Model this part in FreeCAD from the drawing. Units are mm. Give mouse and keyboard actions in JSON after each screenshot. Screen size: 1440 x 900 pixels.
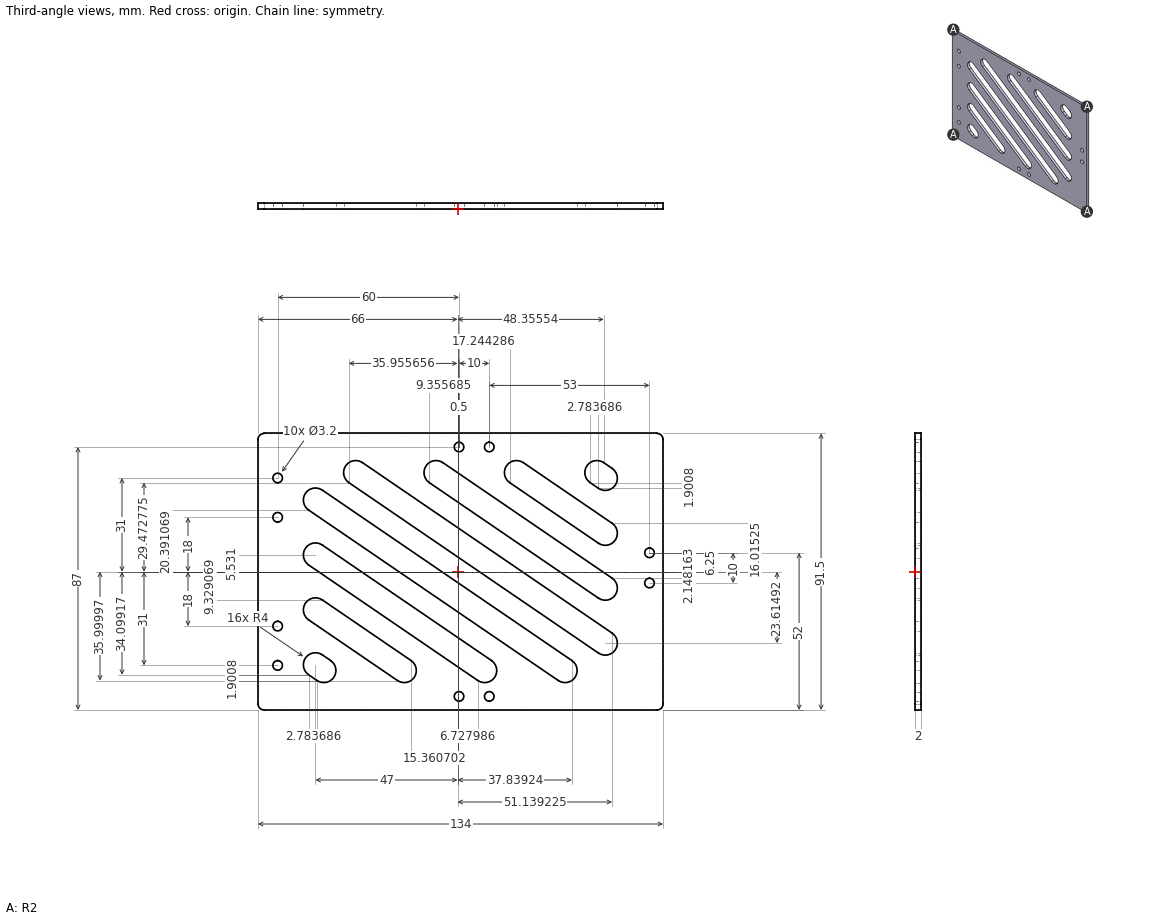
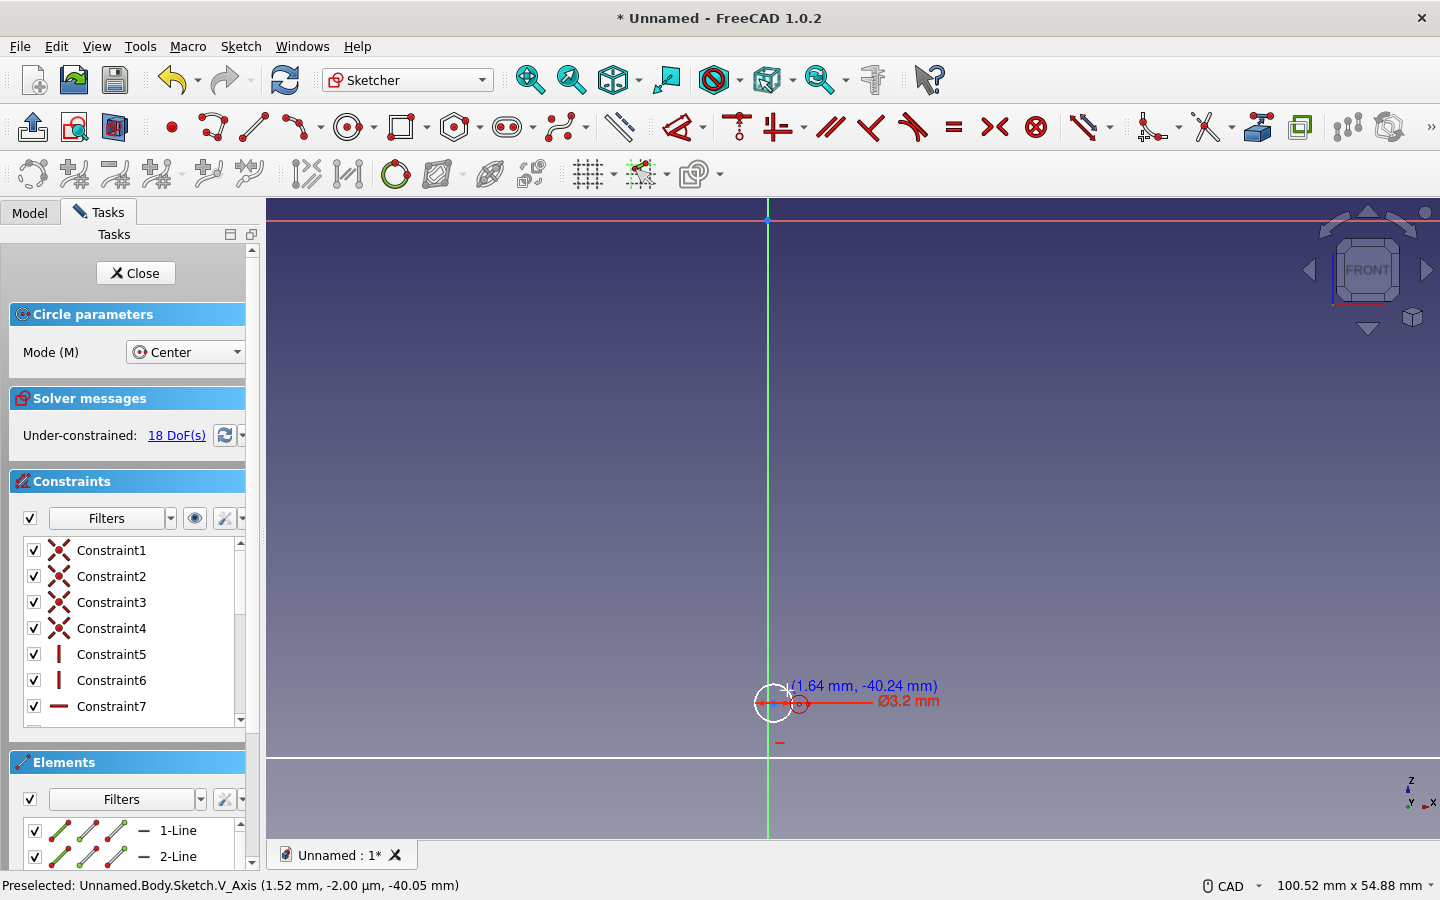
{"action": "scroll", "coordinate": [787, 692], "scroll_direction": "down", "scroll_amount": 5}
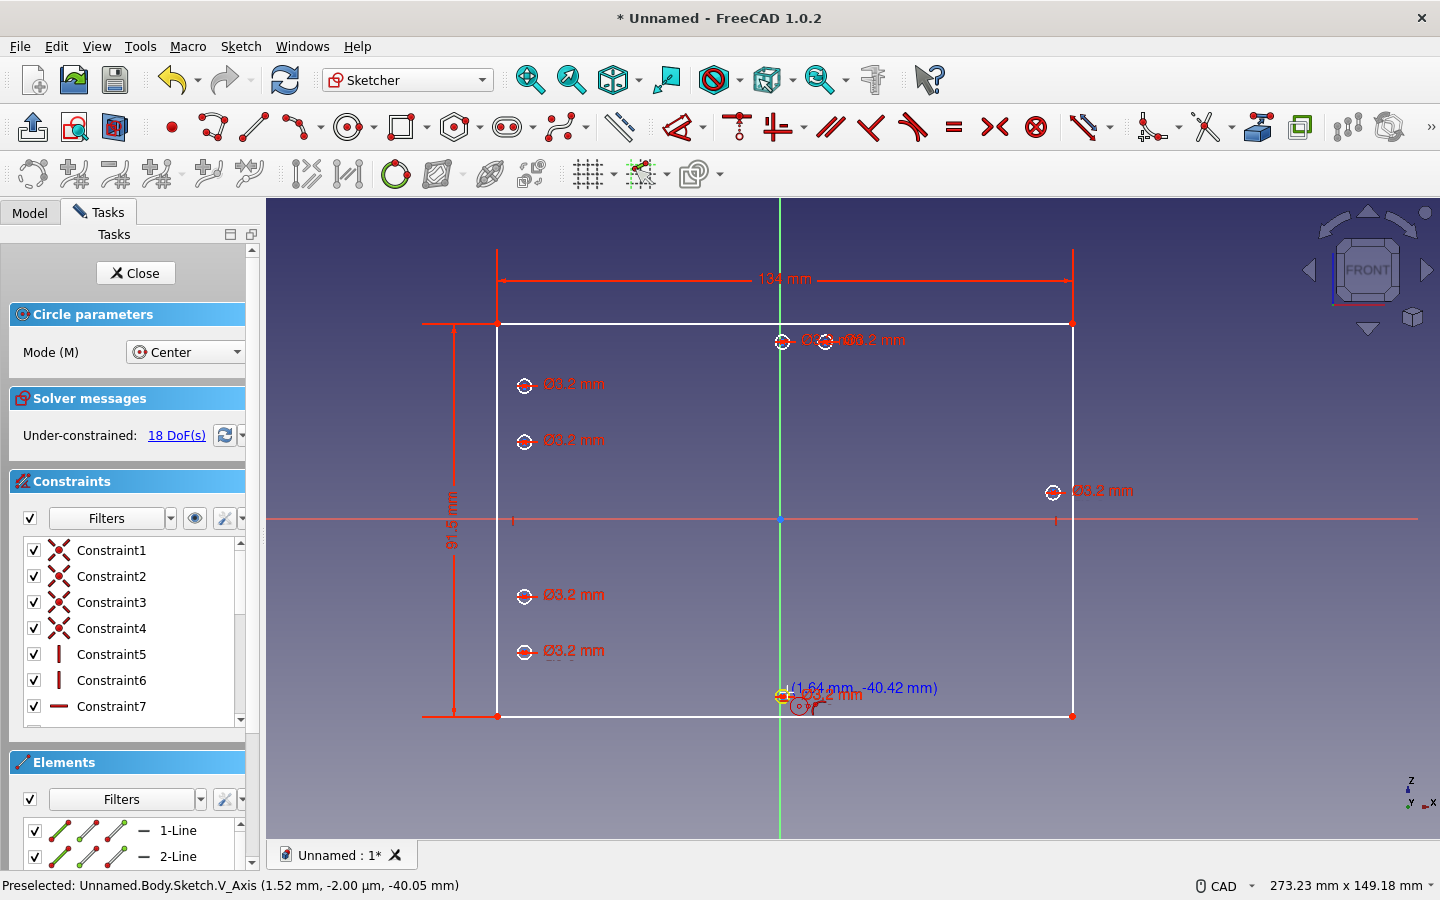
{"action": "scroll", "coordinate": [1053, 535], "scroll_direction": "up", "scroll_amount": 6}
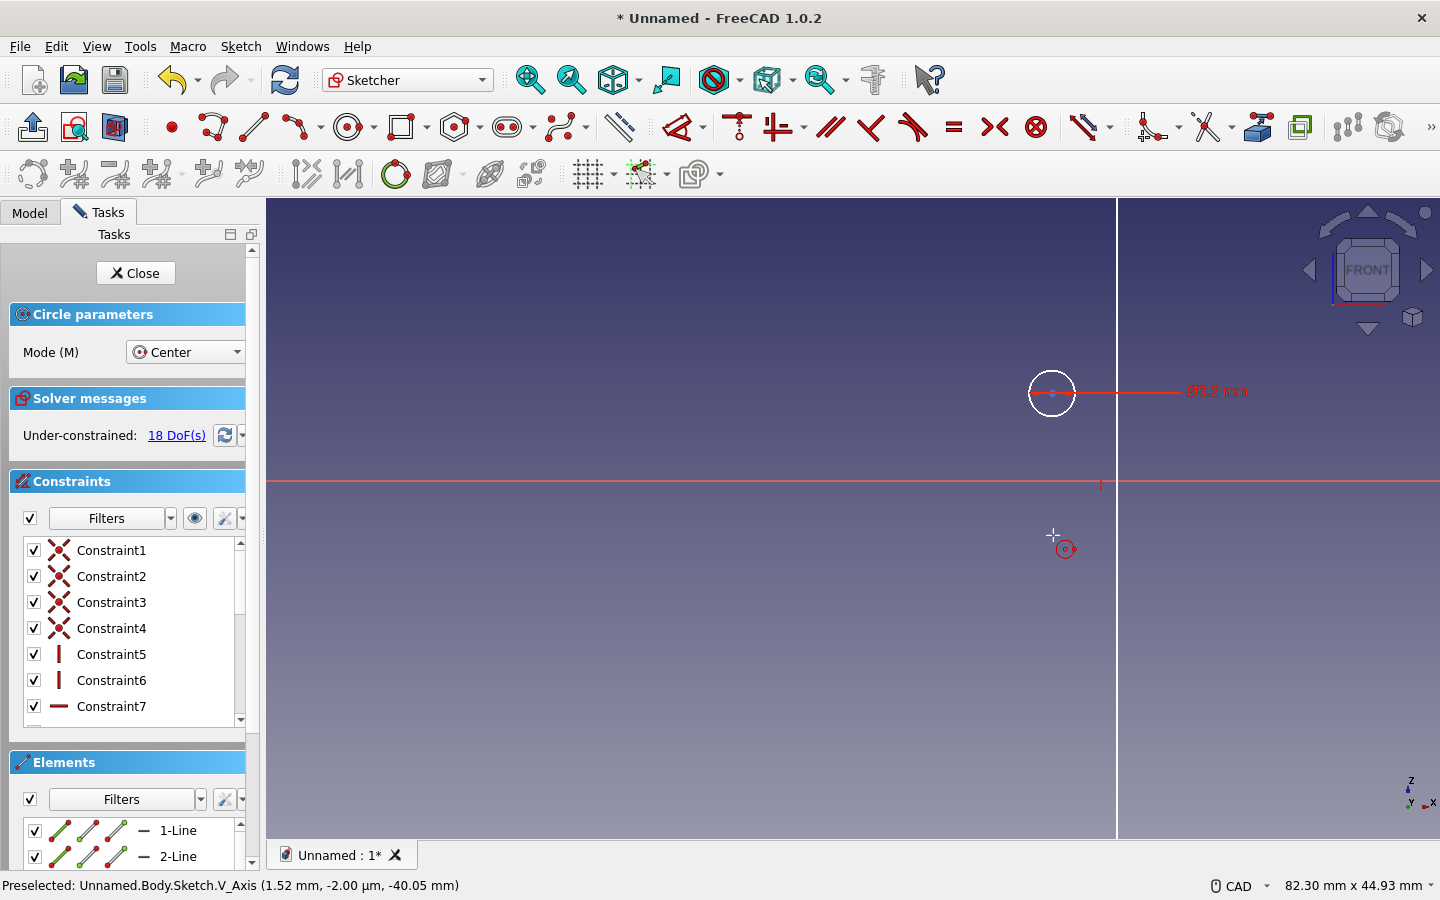
{"action": "left_click", "coordinate": [1052, 535]}
{"action": "mouse_move", "coordinate": [1068, 519]}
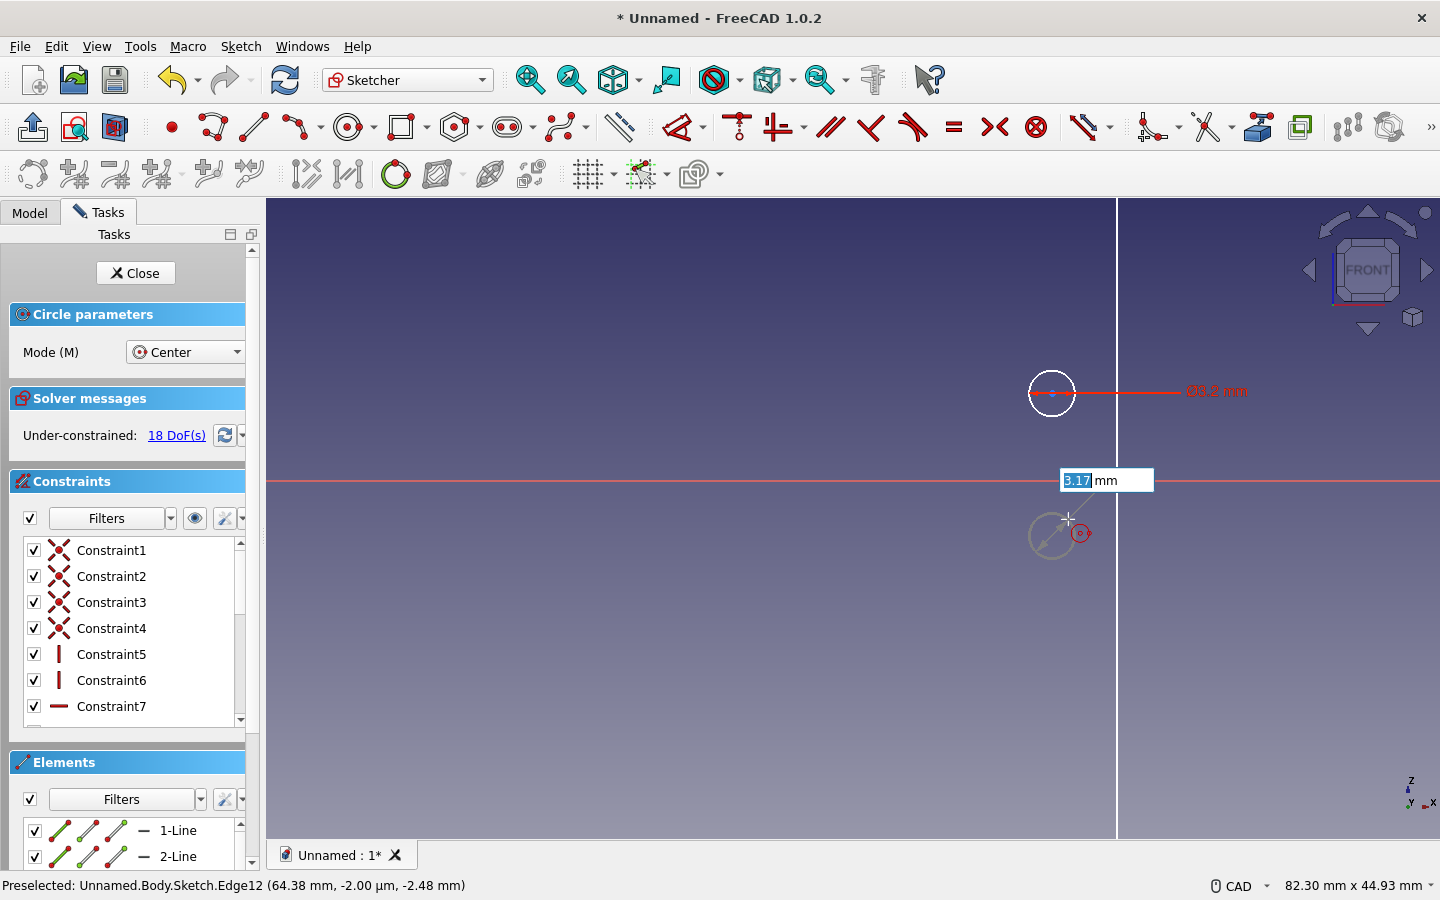
{"action": "type", "text": "3.2"}
{"action": "key", "text": "Return"}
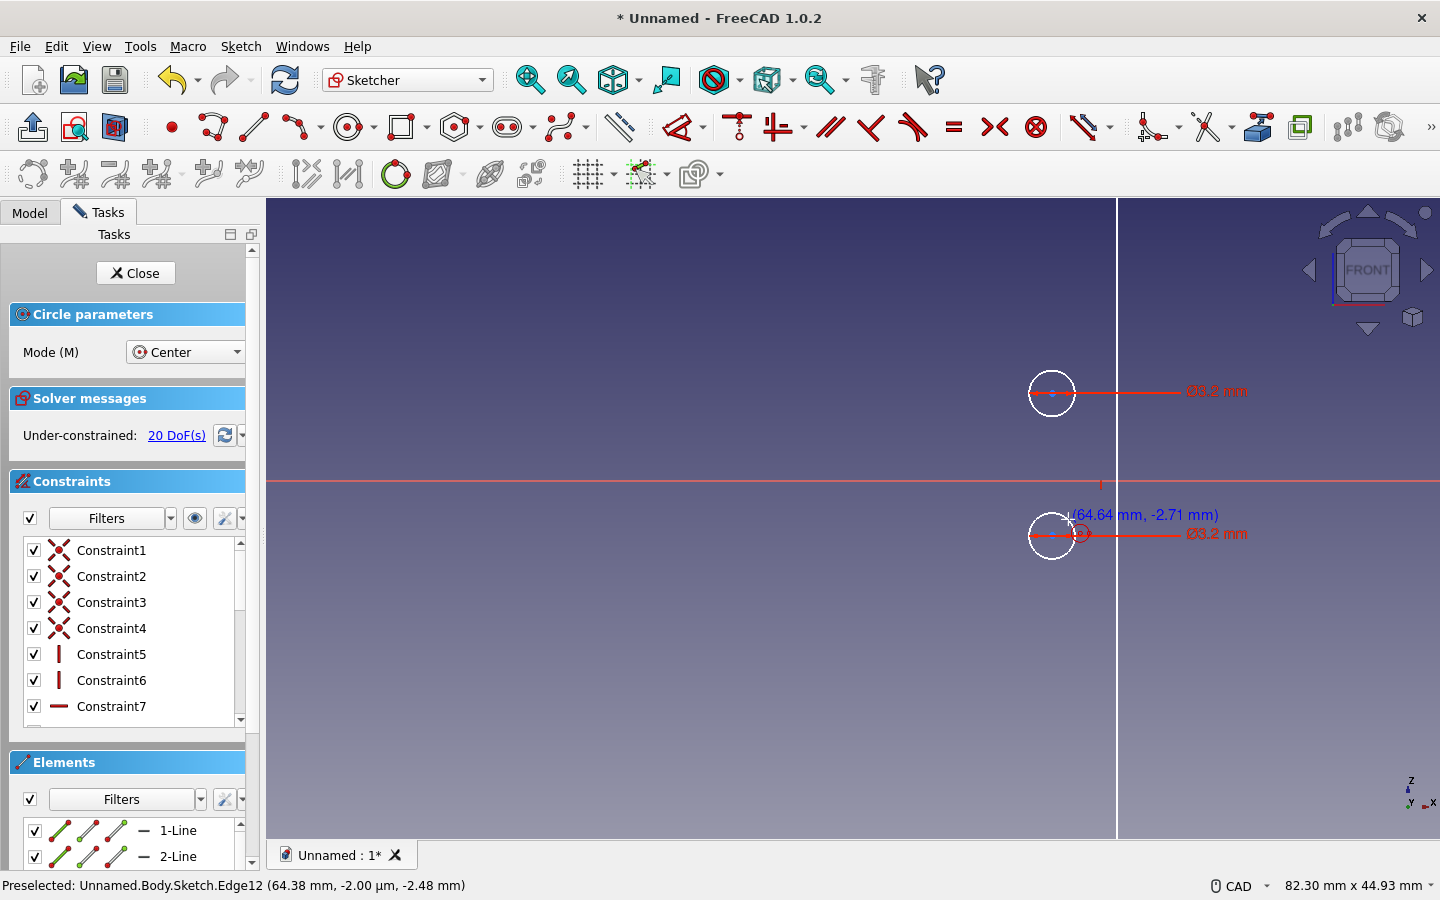
{"action": "scroll", "coordinate": [1054, 535], "scroll_direction": "down", "scroll_amount": 6}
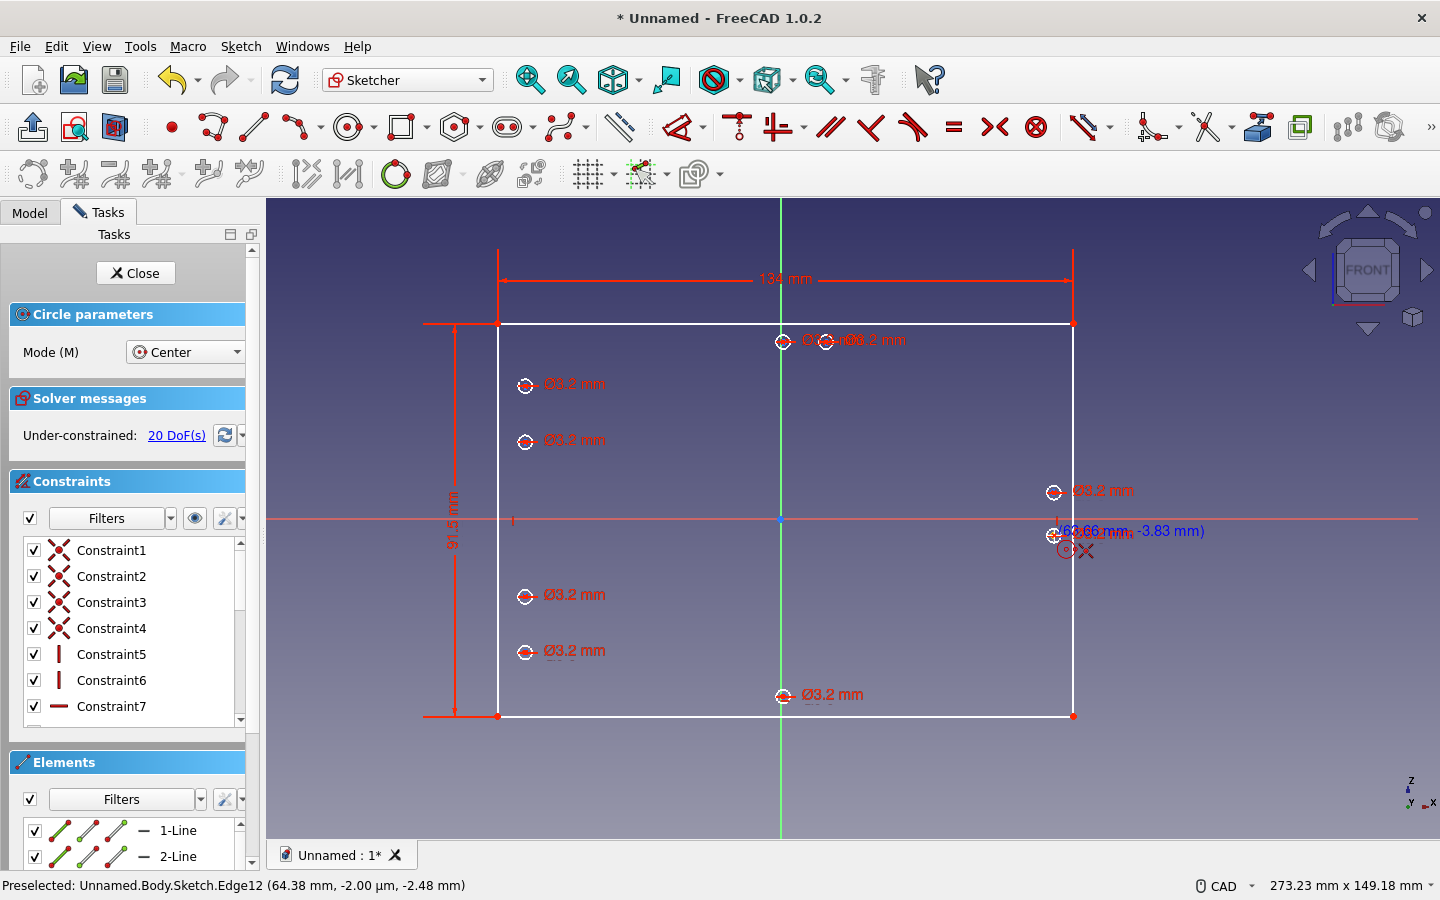
{"action": "scroll", "coordinate": [826, 696], "scroll_direction": "up", "scroll_amount": 6}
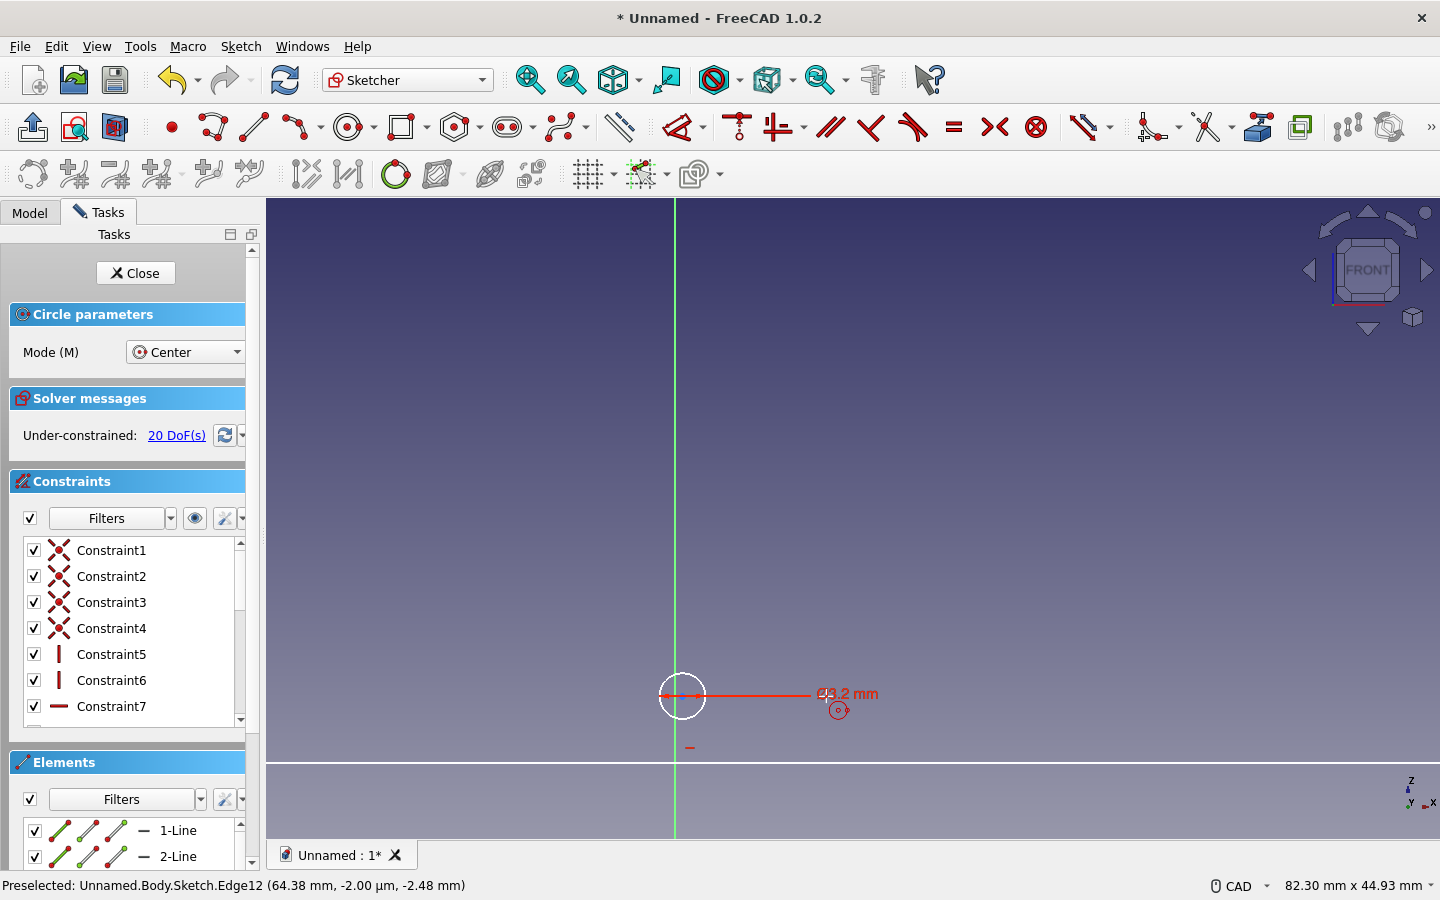
{"action": "left_click", "coordinate": [825, 696]}
{"action": "mouse_move", "coordinate": [841, 680]}